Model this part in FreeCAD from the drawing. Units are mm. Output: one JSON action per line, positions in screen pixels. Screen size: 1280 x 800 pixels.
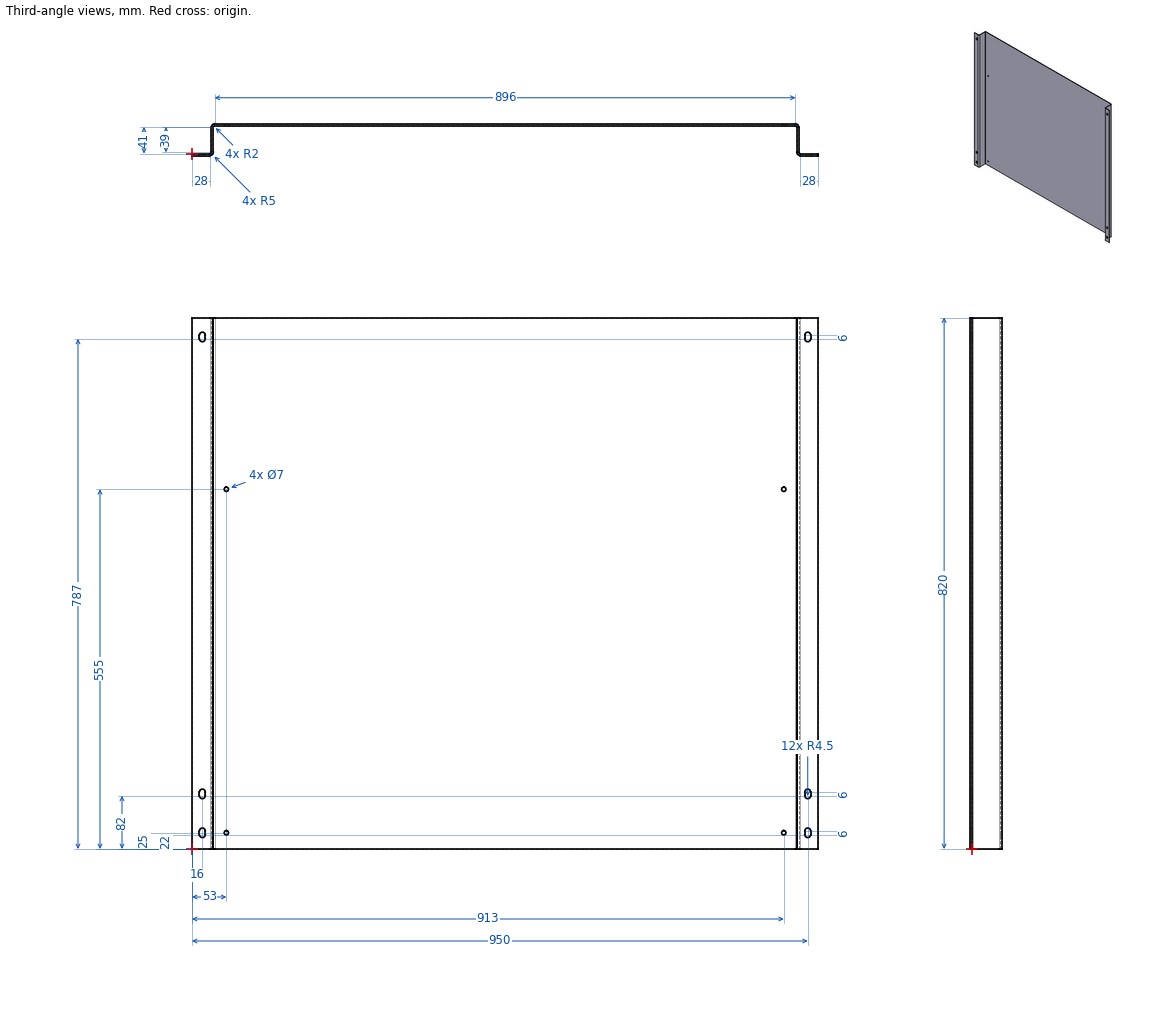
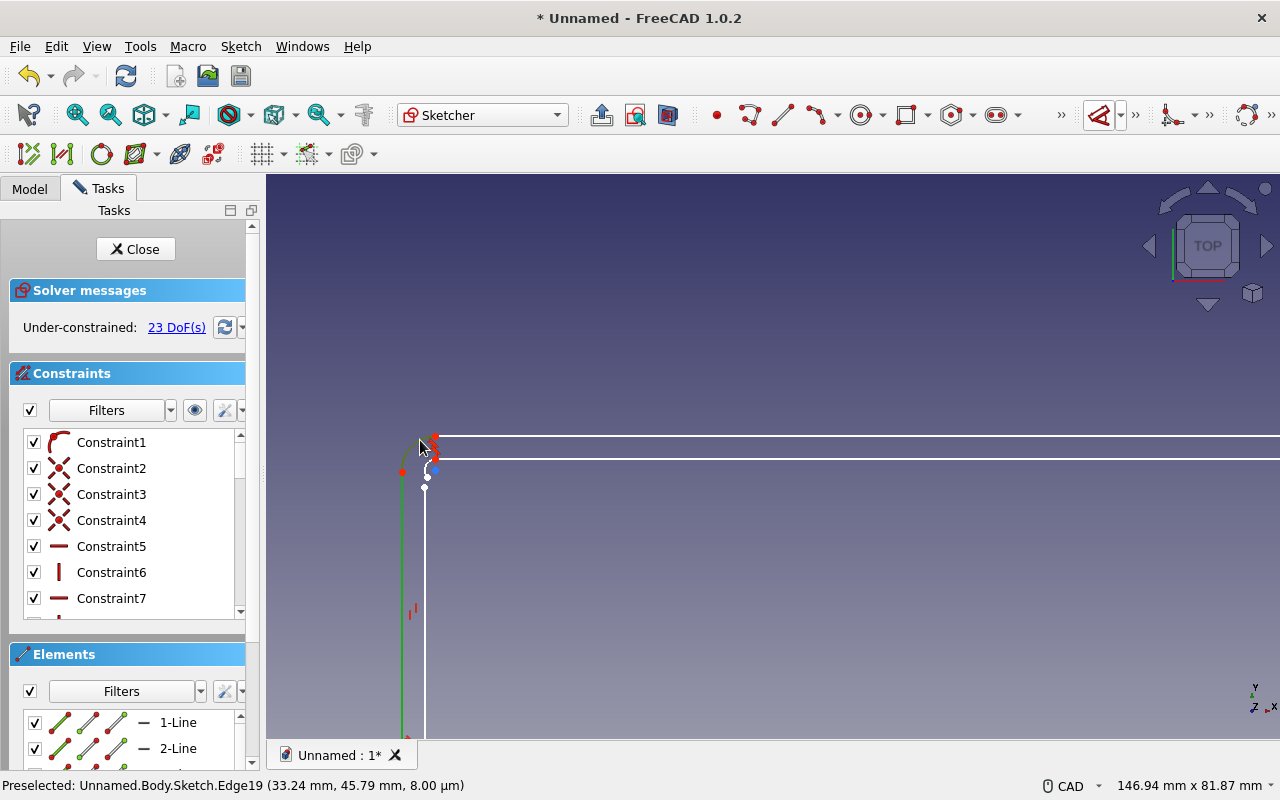
{"action": "key", "text": "t"}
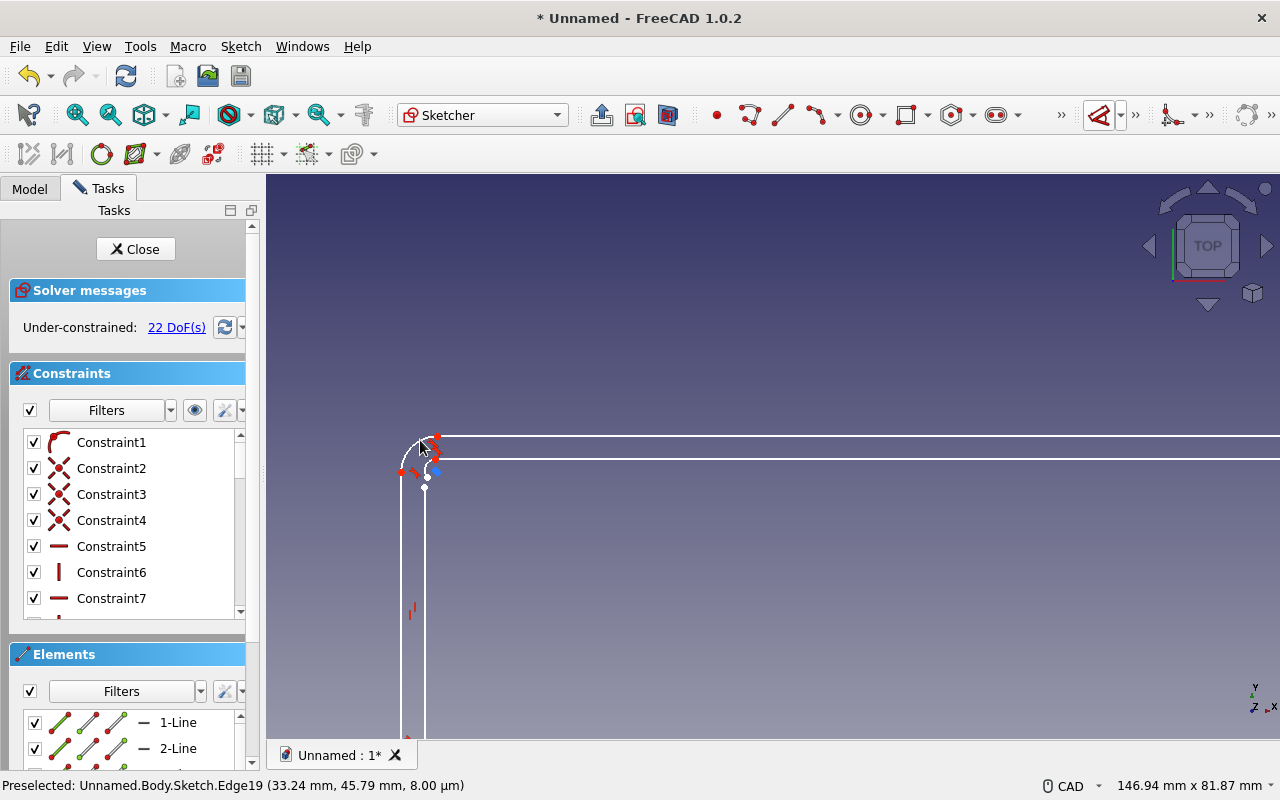
{"action": "left_click", "coordinate": [401, 553]}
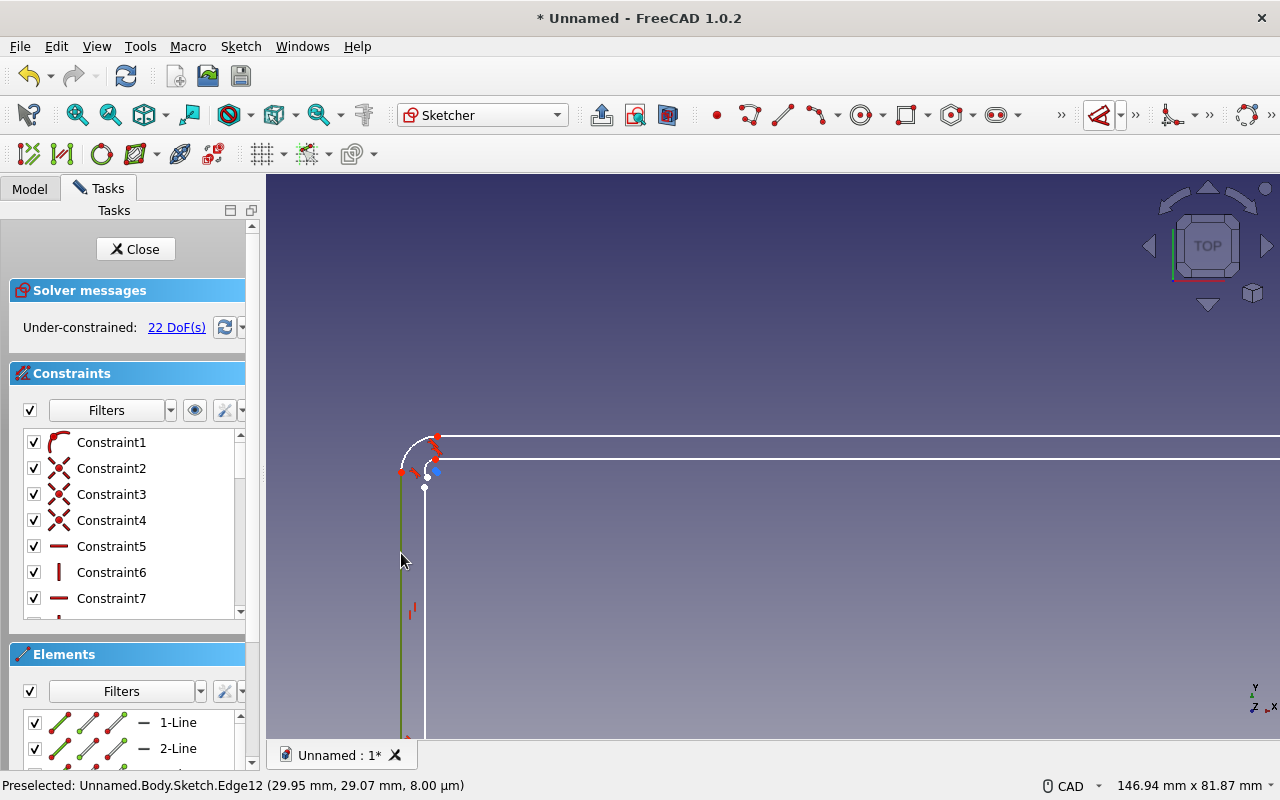
{"action": "scroll", "coordinate": [423, 442], "scroll_direction": "down", "scroll_amount": 12}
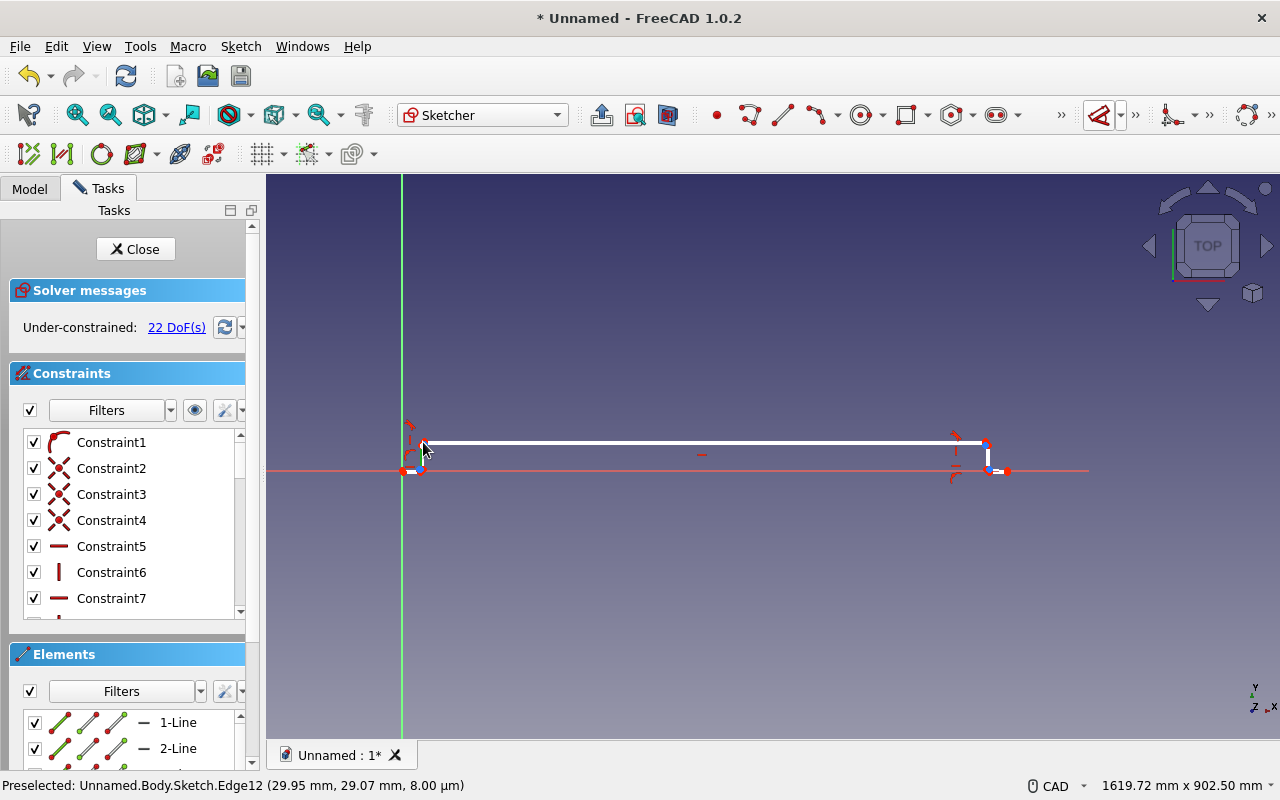
{"action": "scroll", "coordinate": [421, 470], "scroll_direction": "up", "scroll_amount": 14}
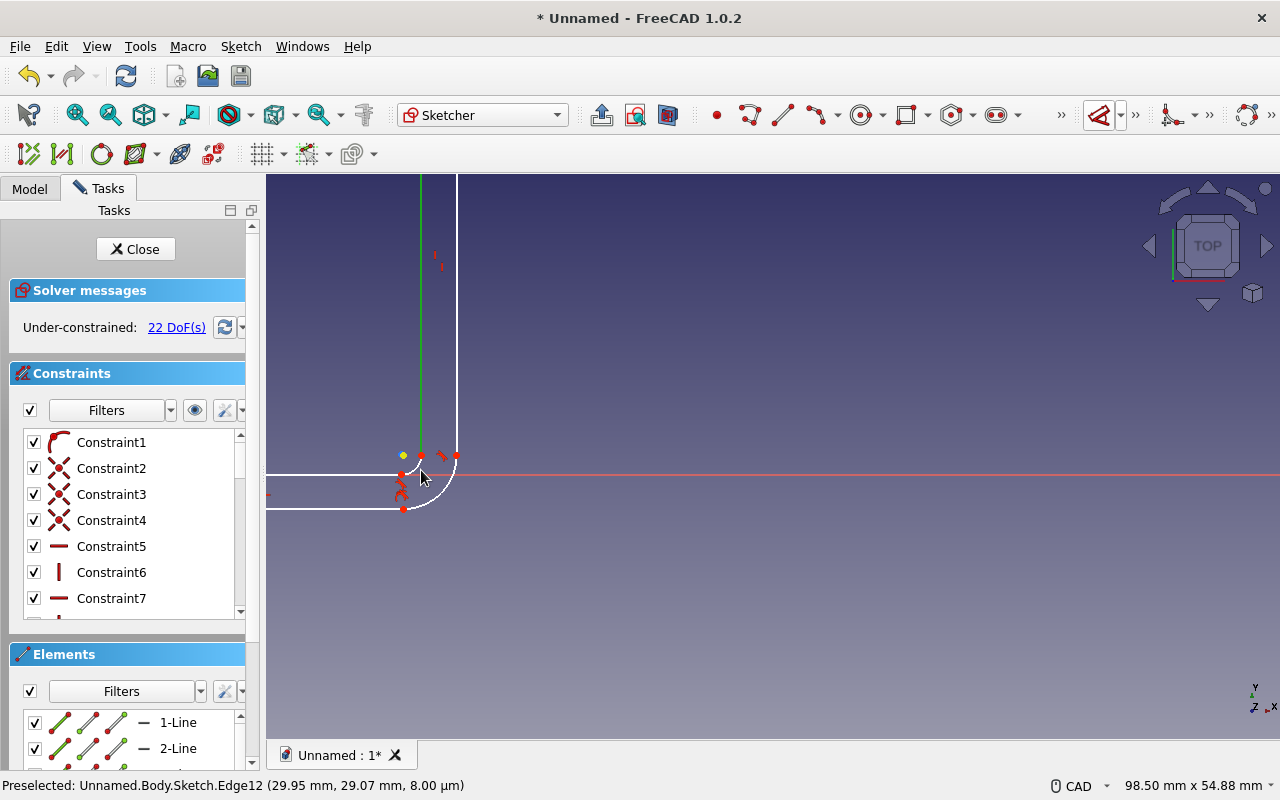
{"action": "left_click", "coordinate": [415, 469]}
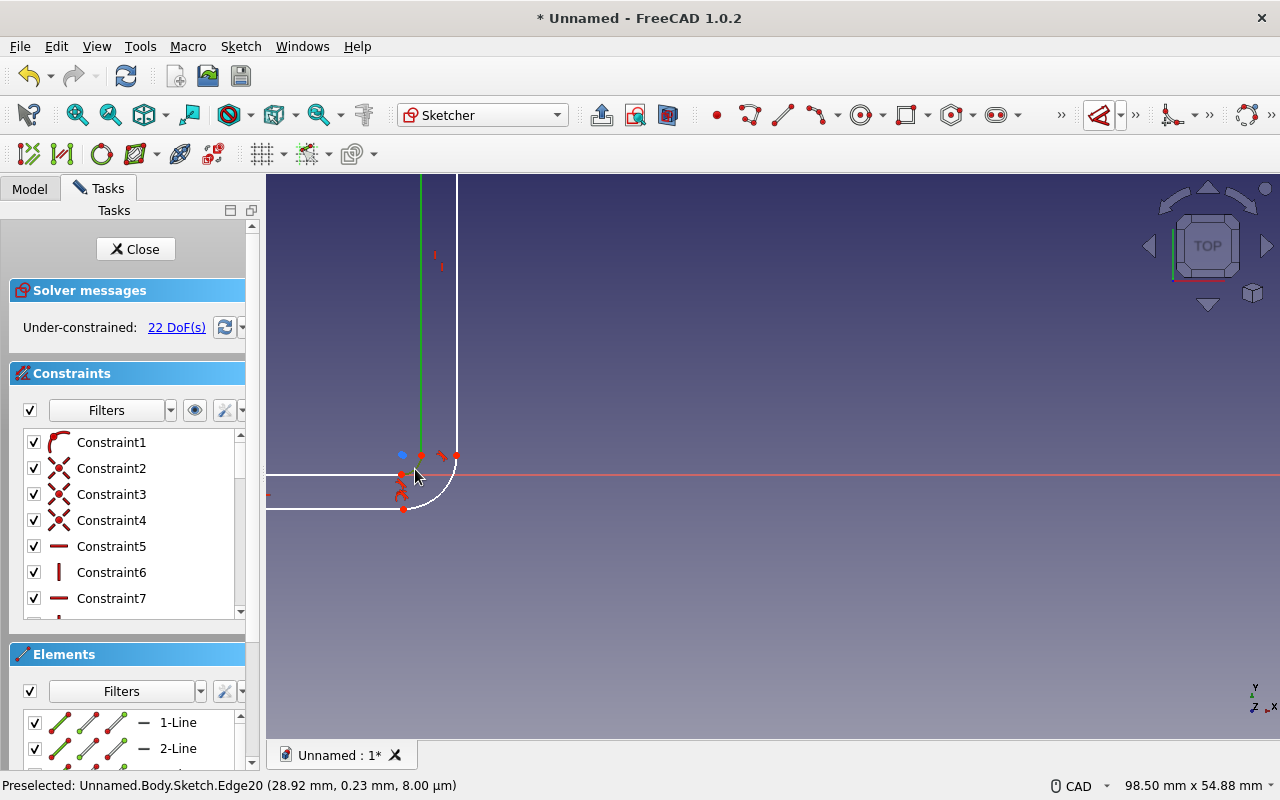
{"action": "key", "text": "t"}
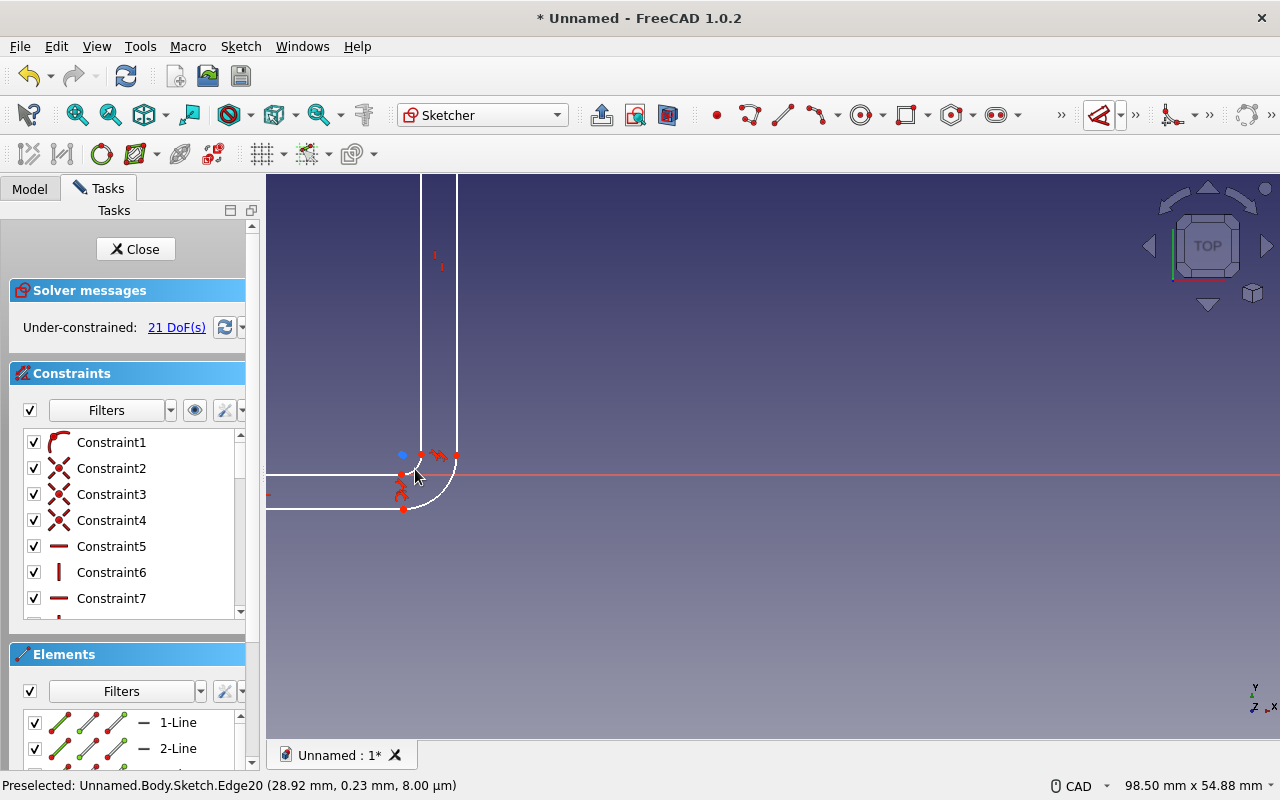
{"action": "scroll", "coordinate": [421, 470], "scroll_direction": "down", "scroll_amount": 14}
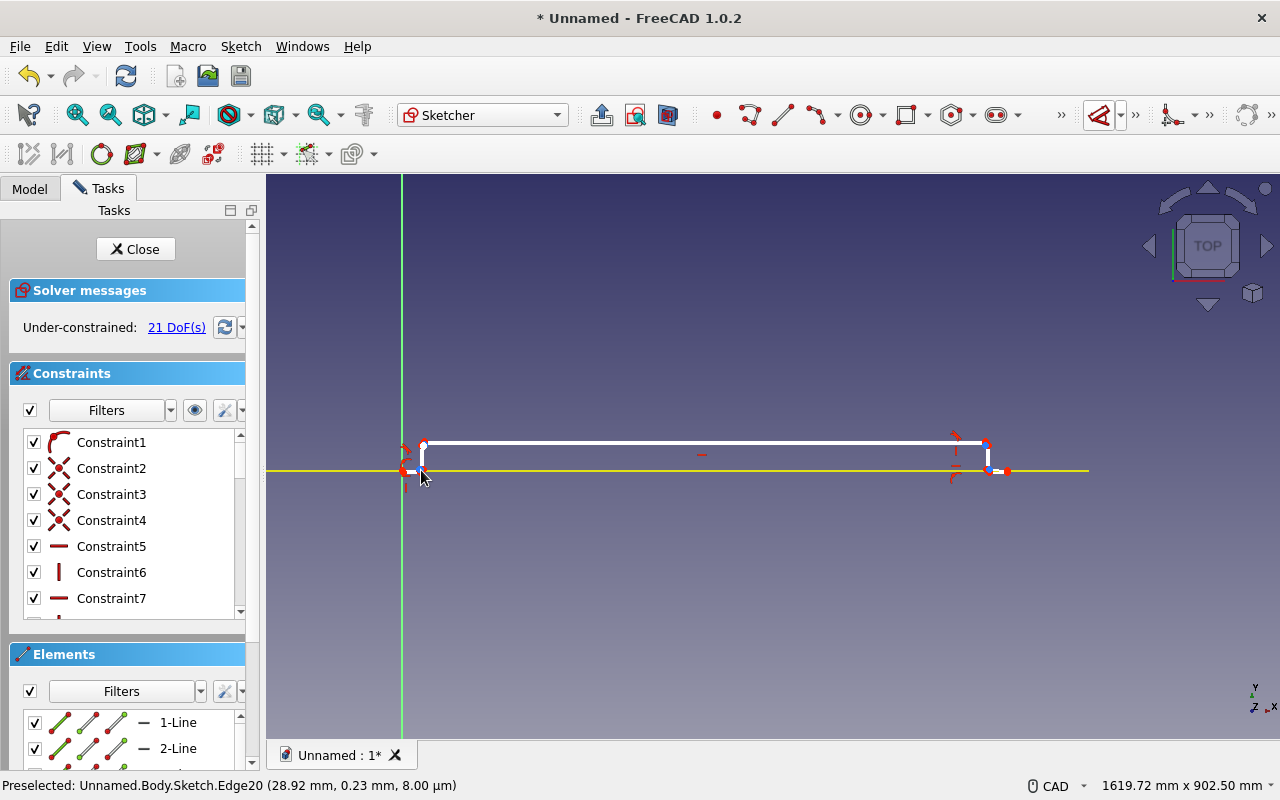
{"action": "scroll", "coordinate": [403, 472], "scroll_direction": "up", "scroll_amount": 14}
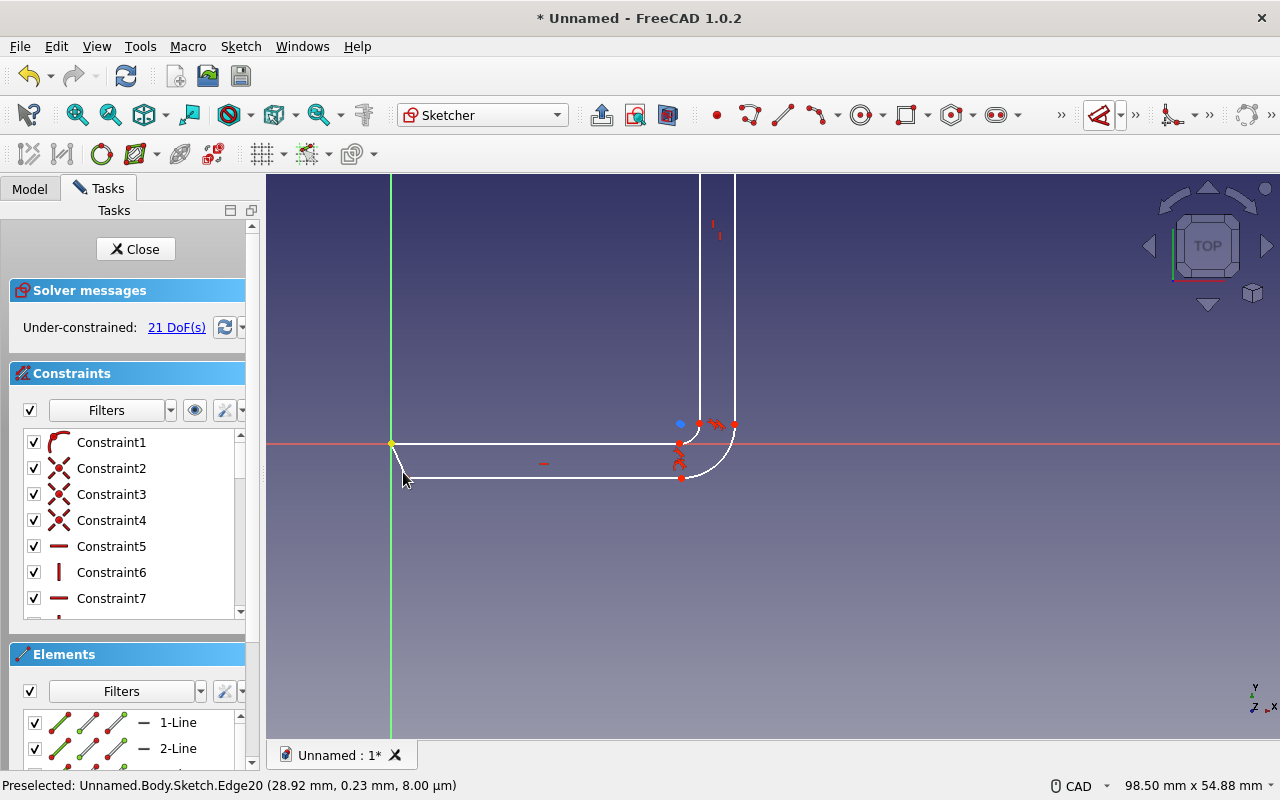
{"action": "left_click", "coordinate": [402, 468]}